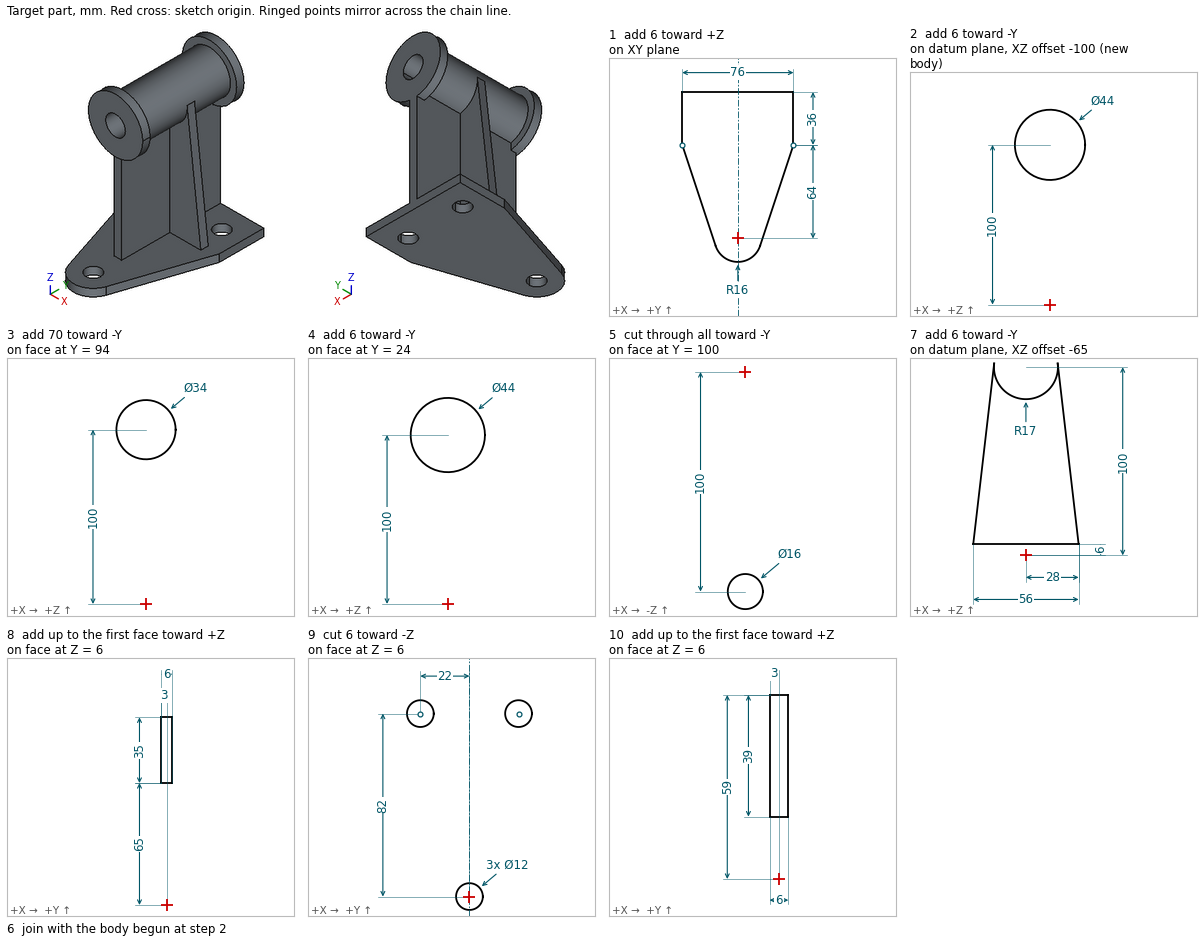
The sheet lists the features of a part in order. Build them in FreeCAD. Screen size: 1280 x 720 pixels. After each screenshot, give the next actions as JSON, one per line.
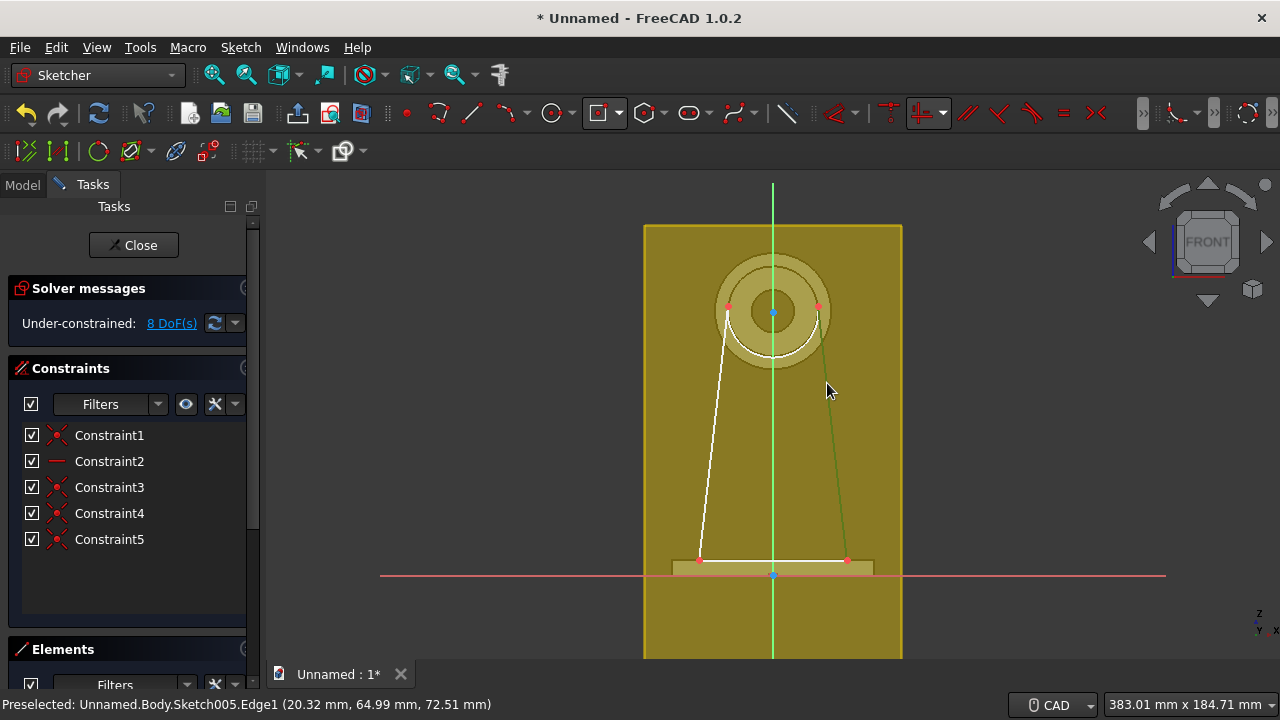
{"action": "left_click", "coordinate": [745, 348]}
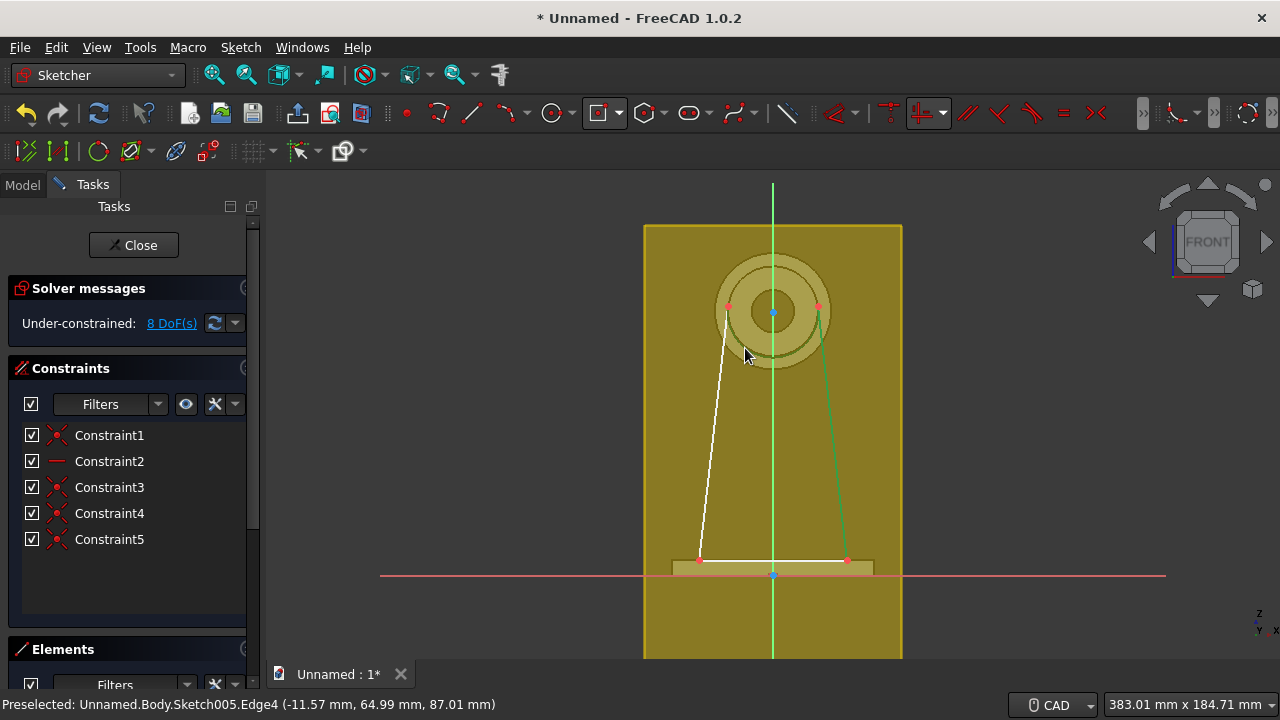
{"action": "left_click", "coordinate": [1032, 114]}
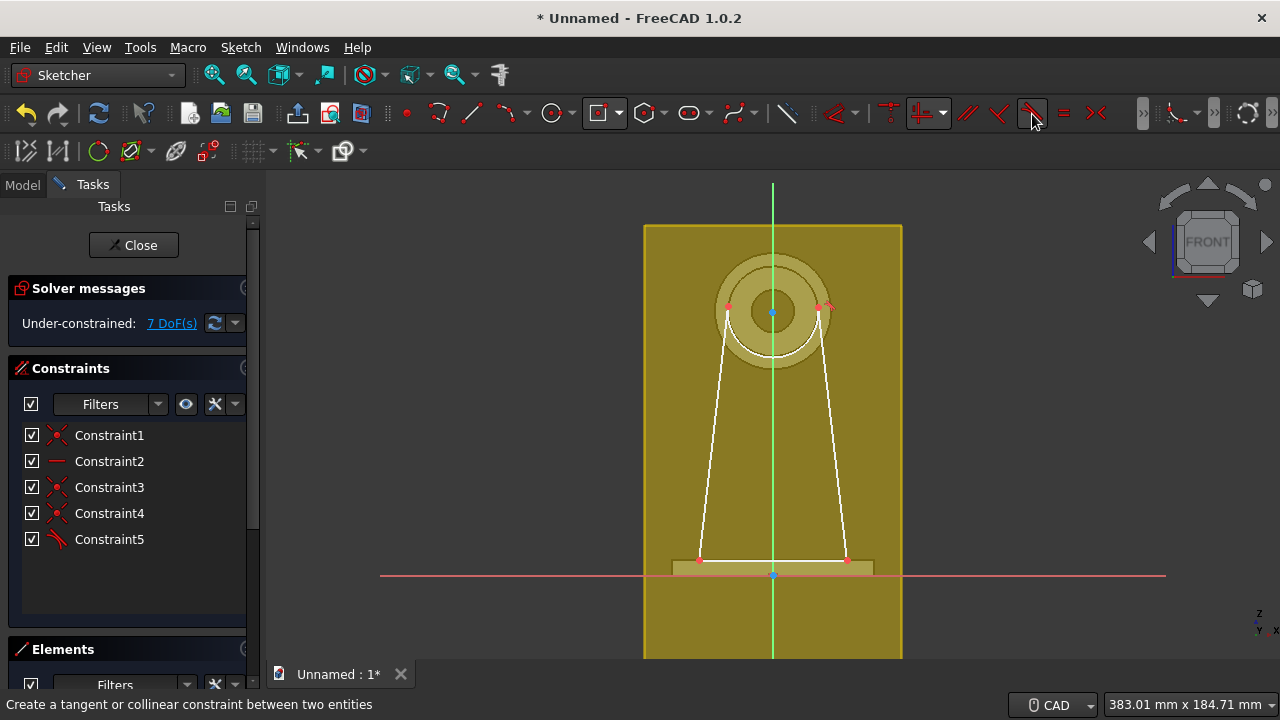
{"action": "left_click", "coordinate": [708, 485]}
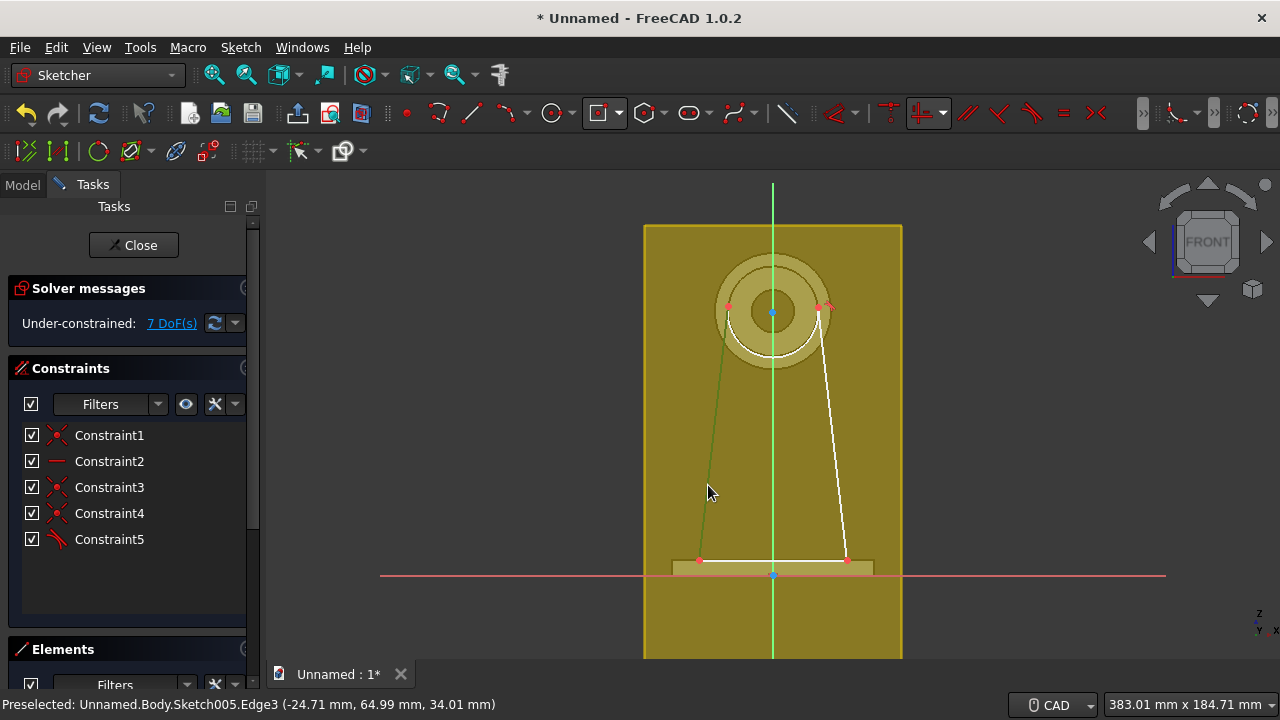
{"action": "left_click", "coordinate": [745, 348]}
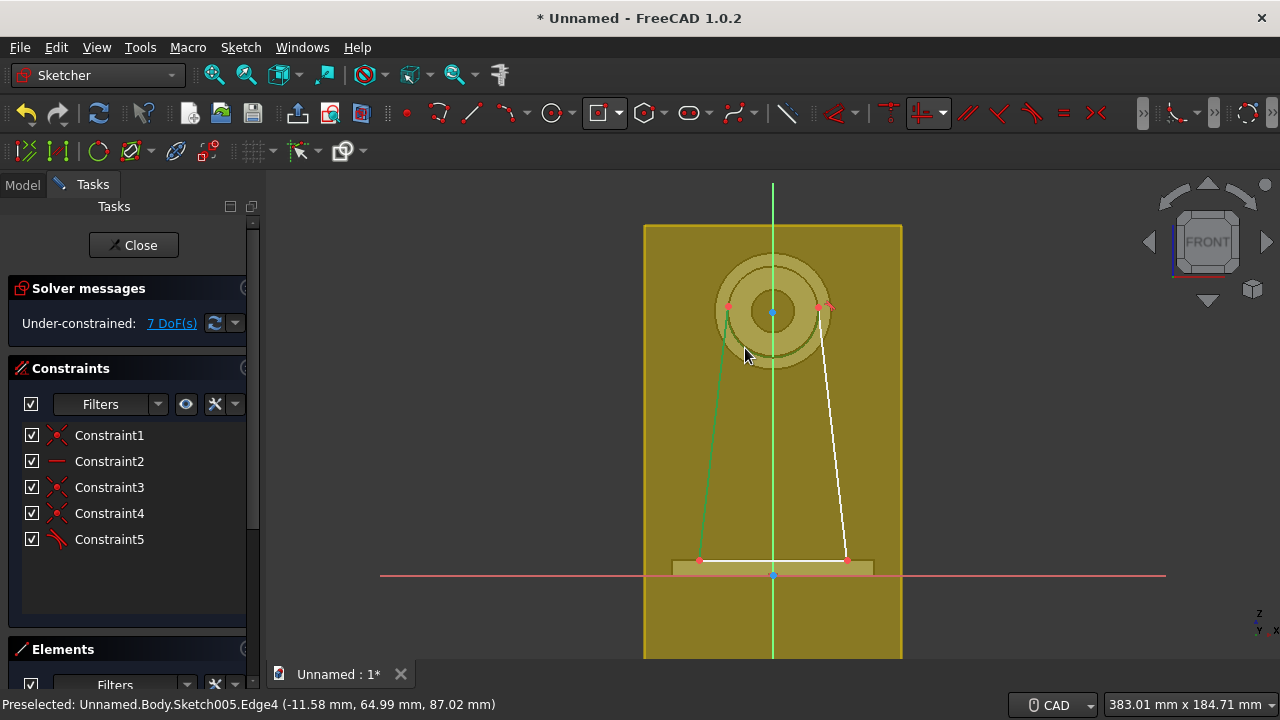
{"action": "left_click", "coordinate": [1032, 114]}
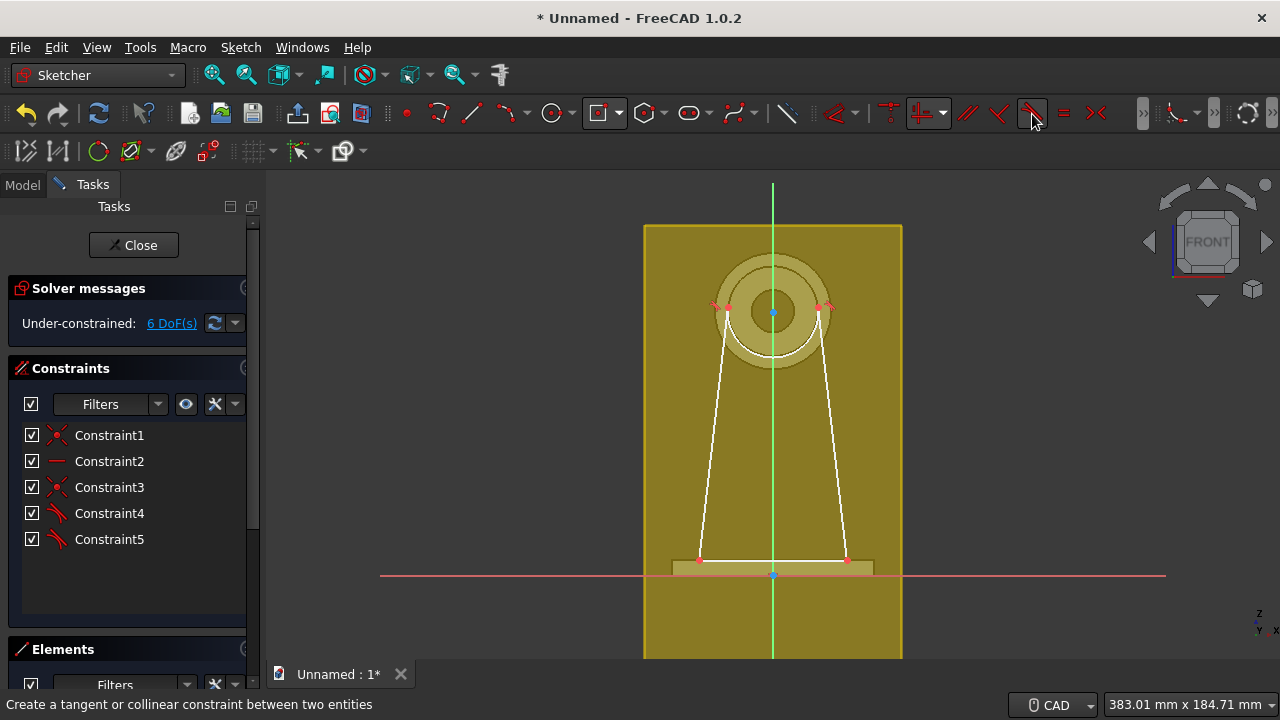
{"action": "left_click", "coordinate": [773, 312]}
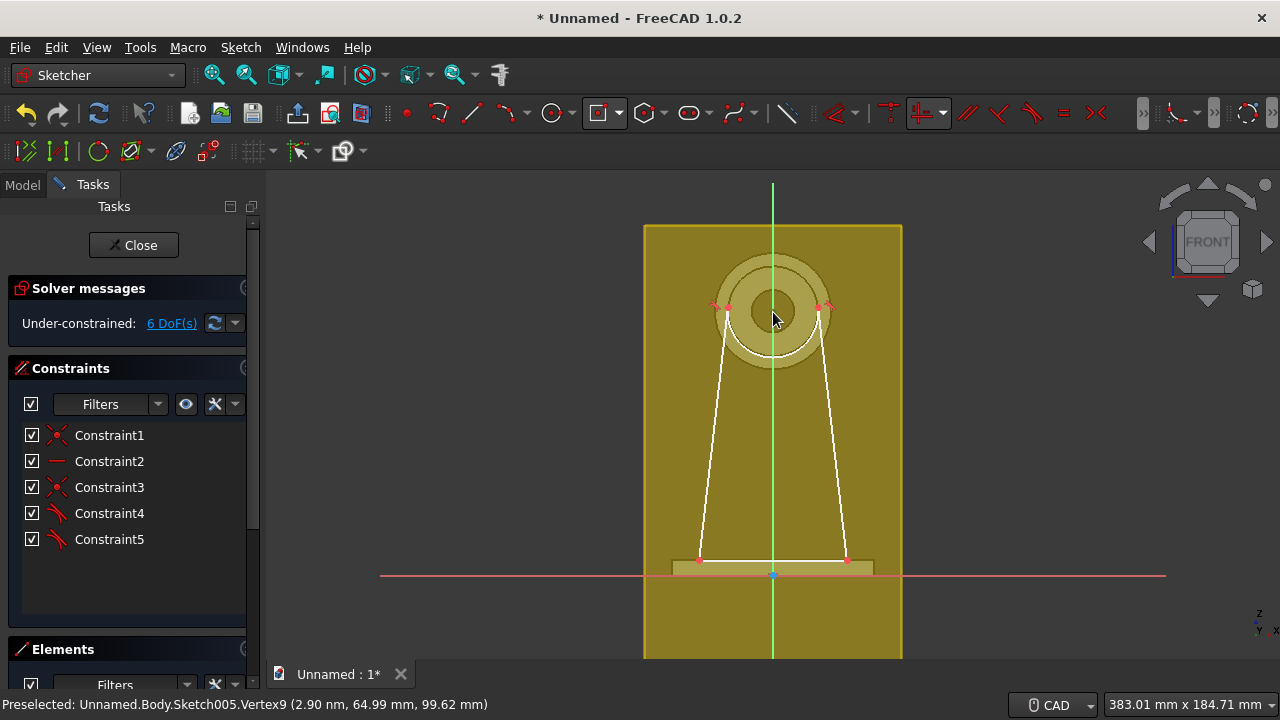
{"action": "left_click", "coordinate": [773, 507]}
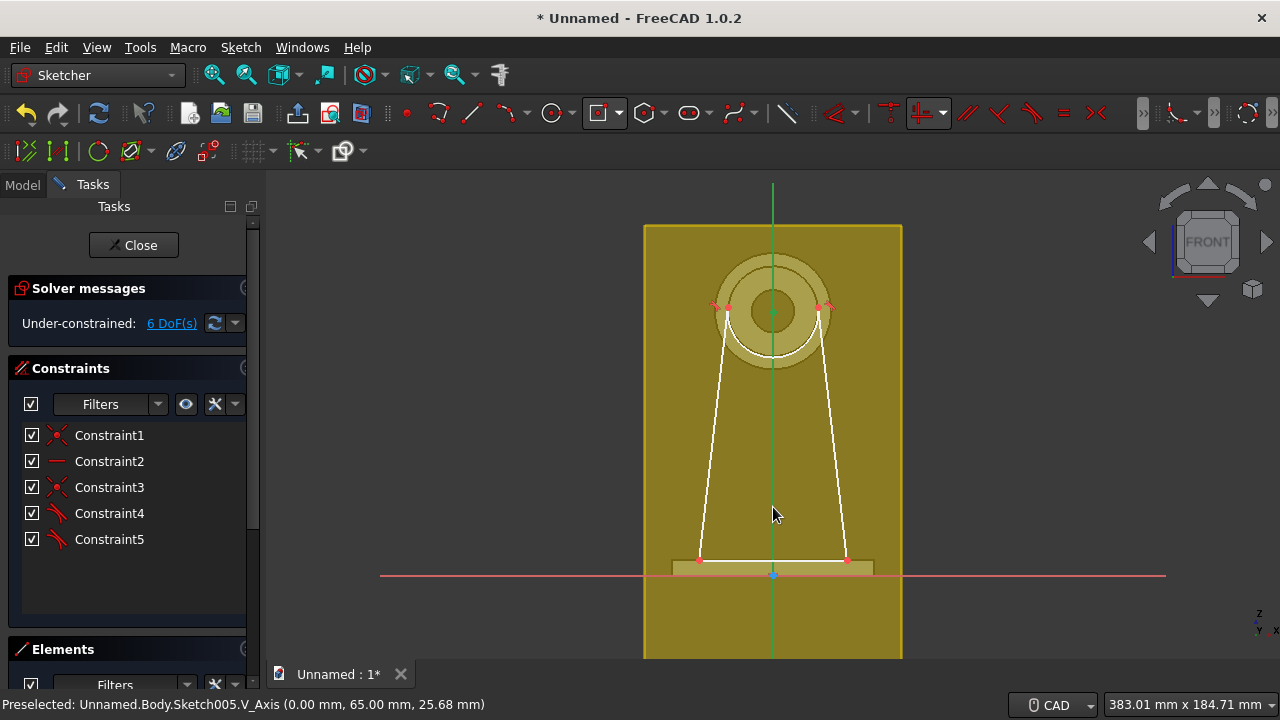
{"action": "key", "text": "c"}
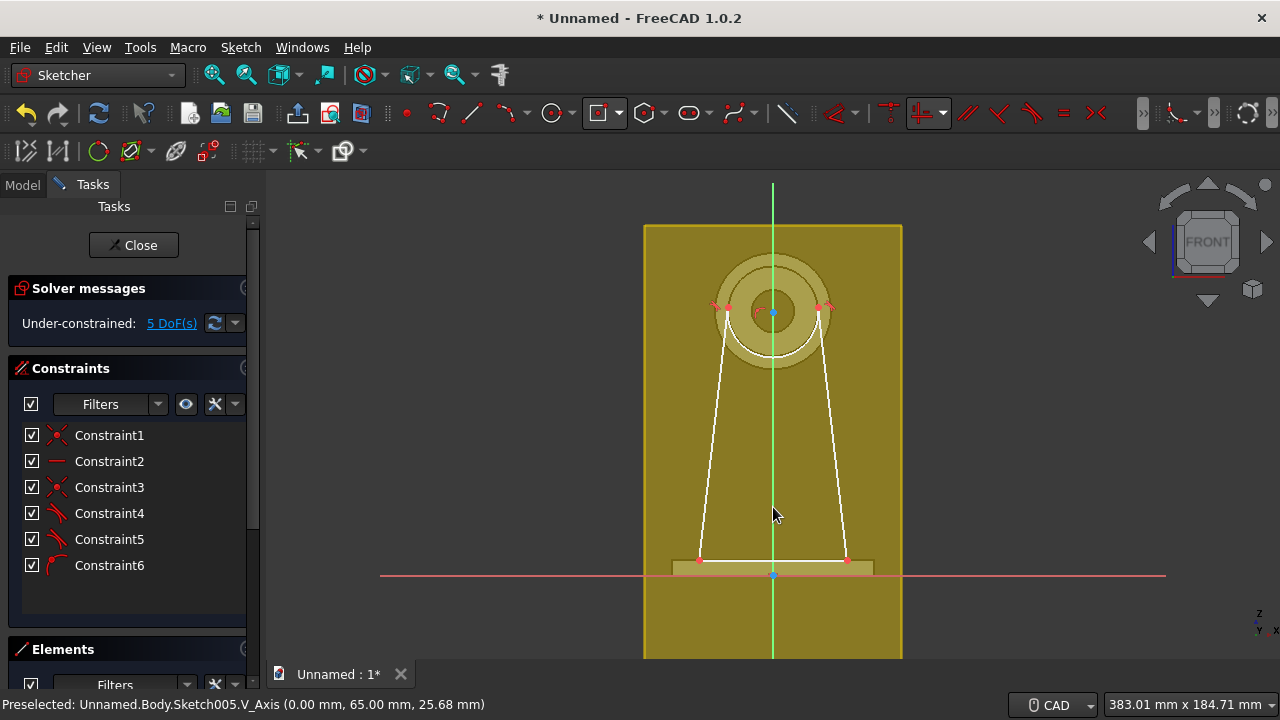
{"action": "left_click", "coordinate": [834, 114]}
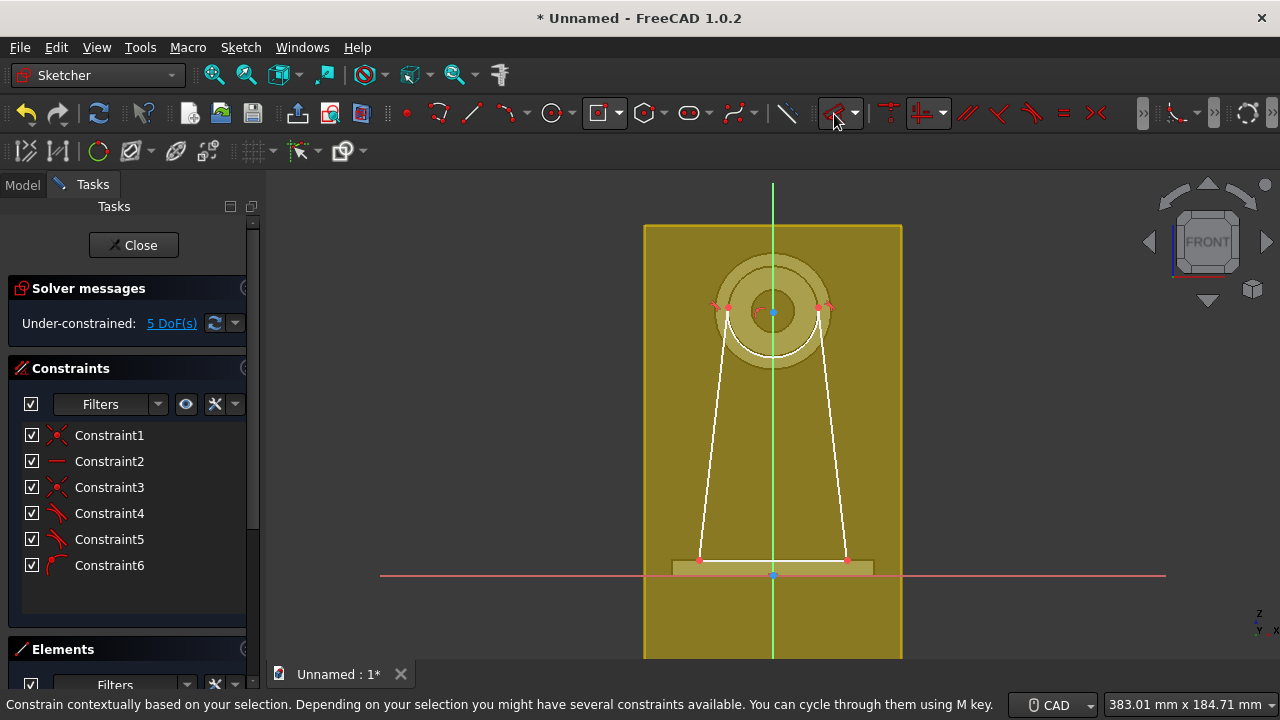
{"action": "left_click", "coordinate": [745, 348]}
{"action": "left_click", "coordinate": [702, 343]}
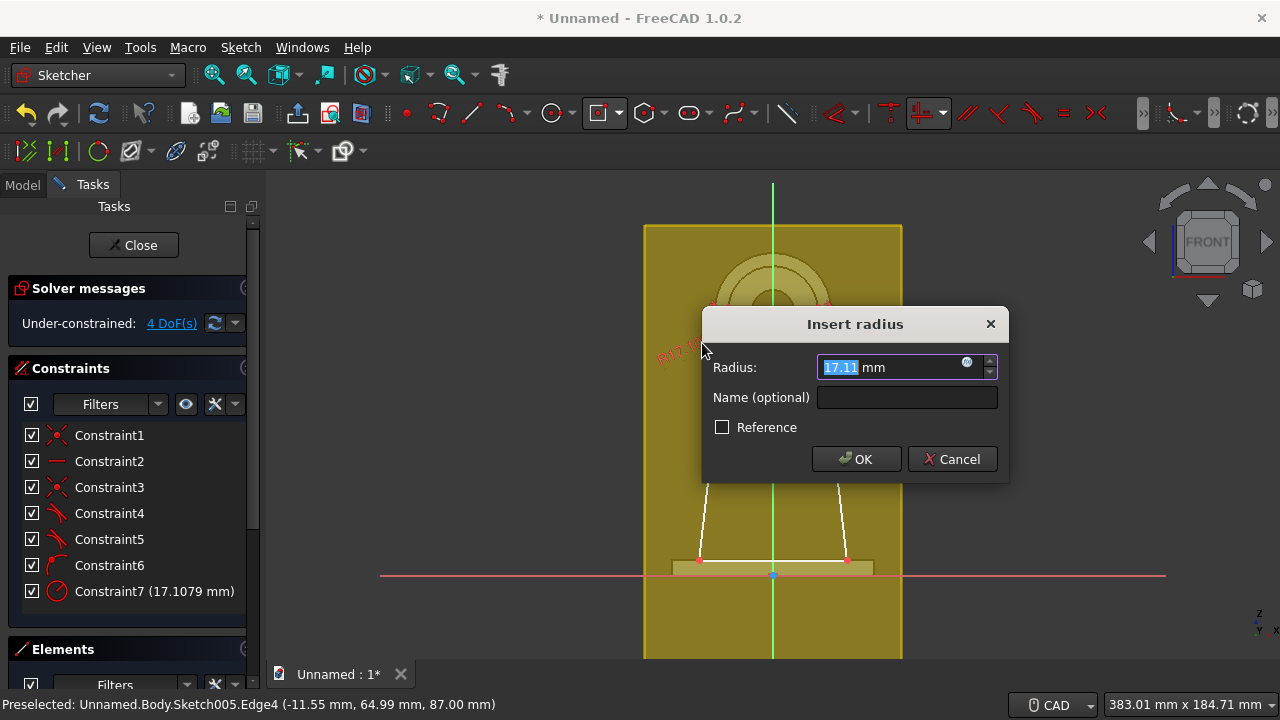
{"action": "type", "text": "17"}
{"action": "key", "text": "Return"}